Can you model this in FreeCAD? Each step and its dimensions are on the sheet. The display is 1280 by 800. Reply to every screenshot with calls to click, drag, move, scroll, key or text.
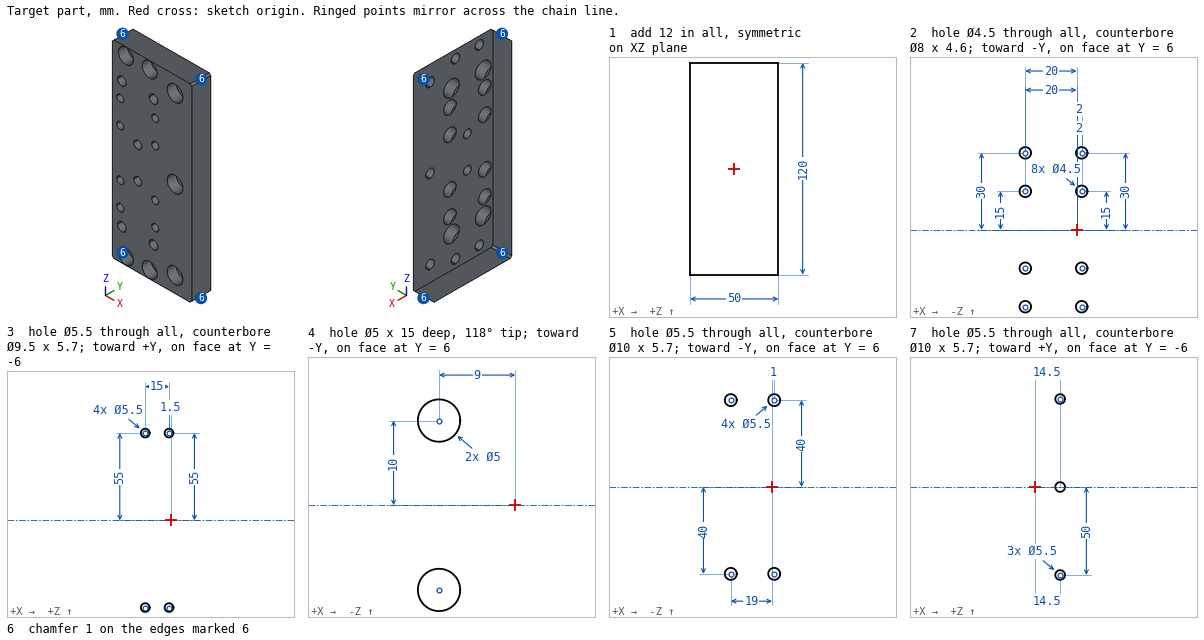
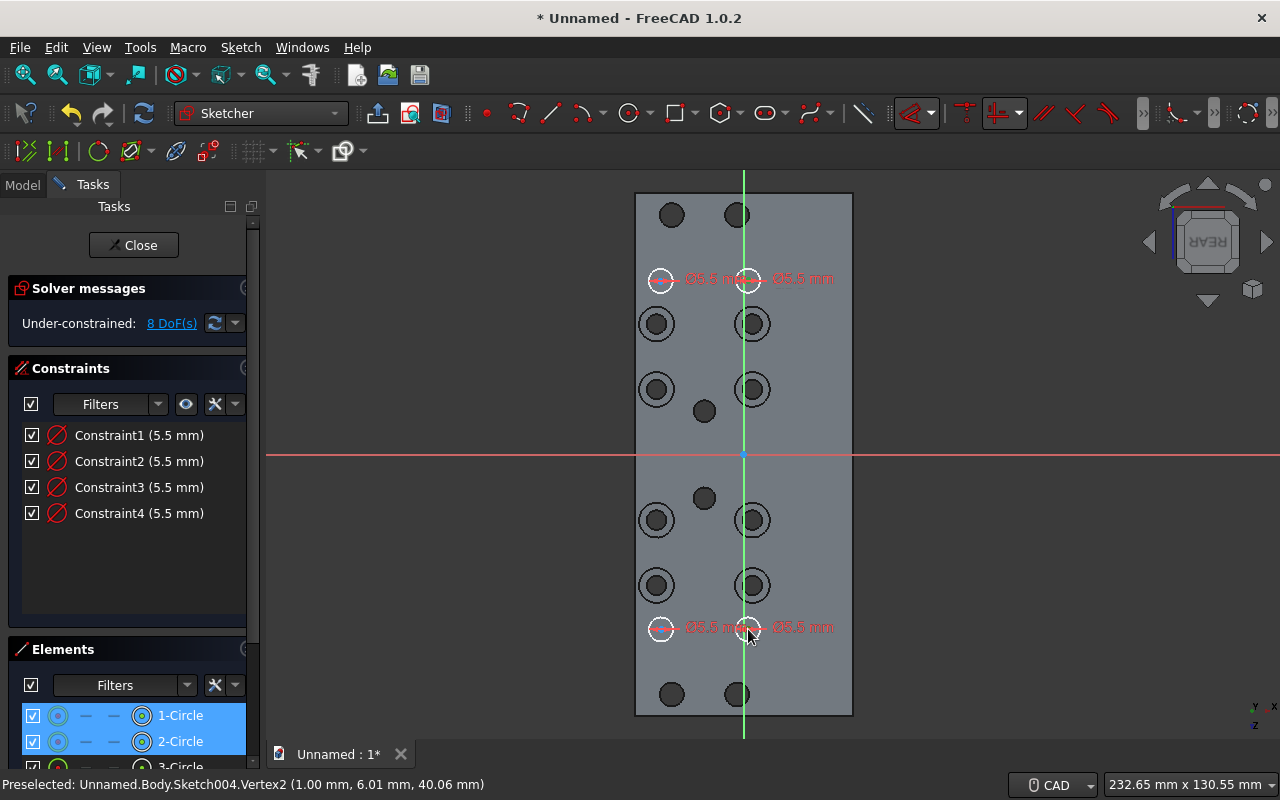
click(353, 455)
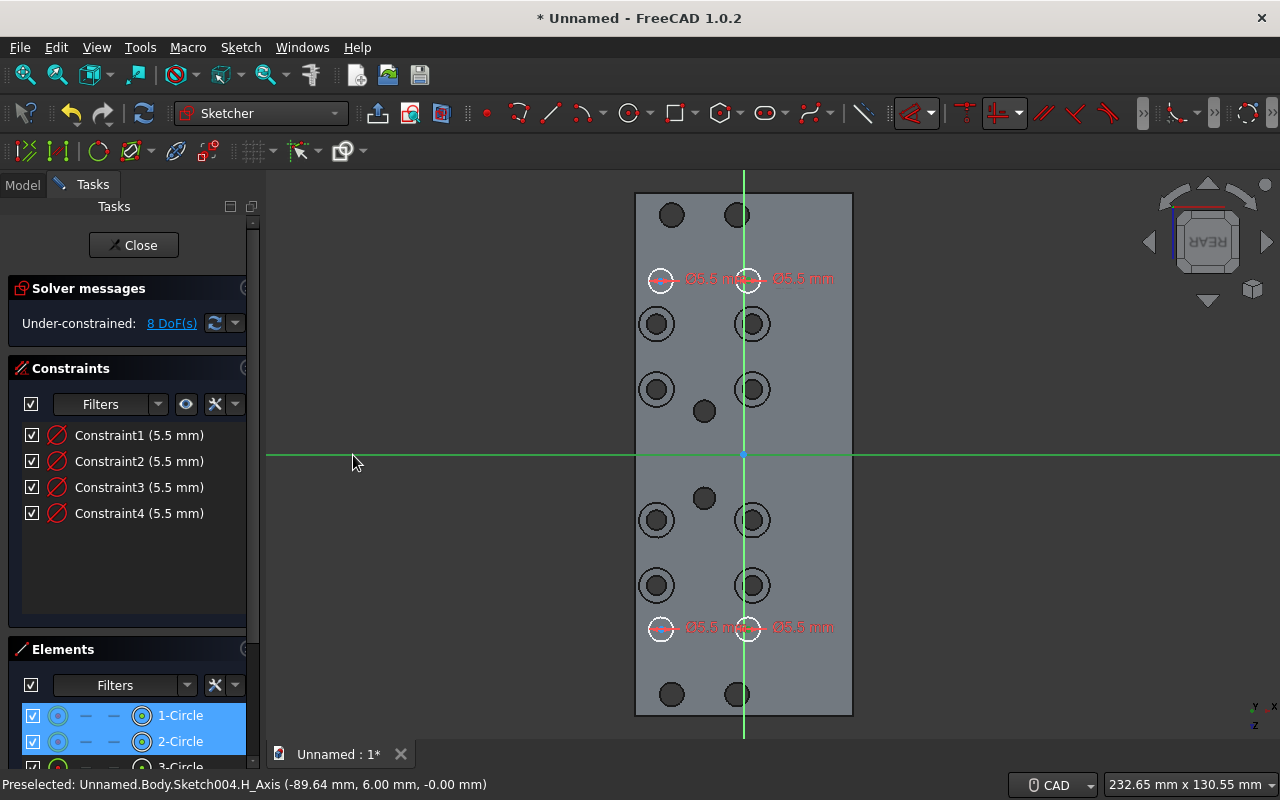
key(s)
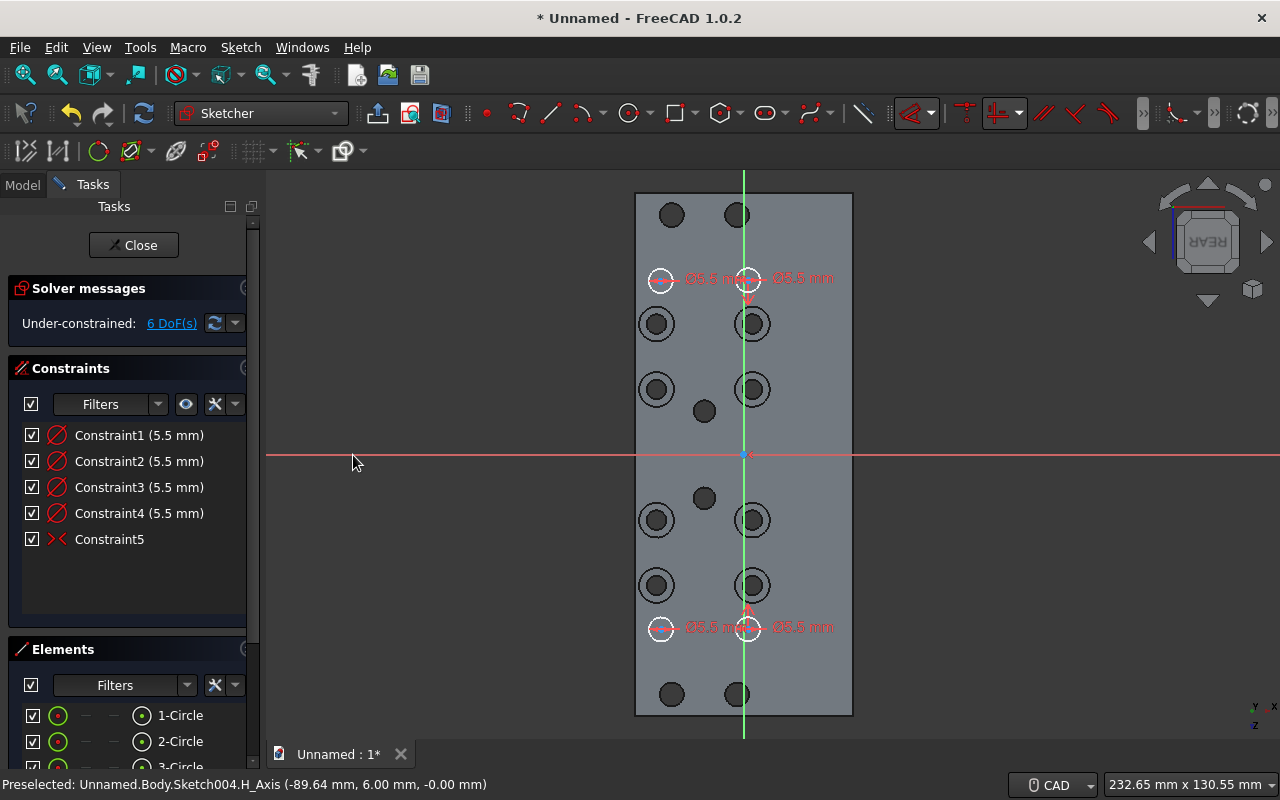
click(661, 629)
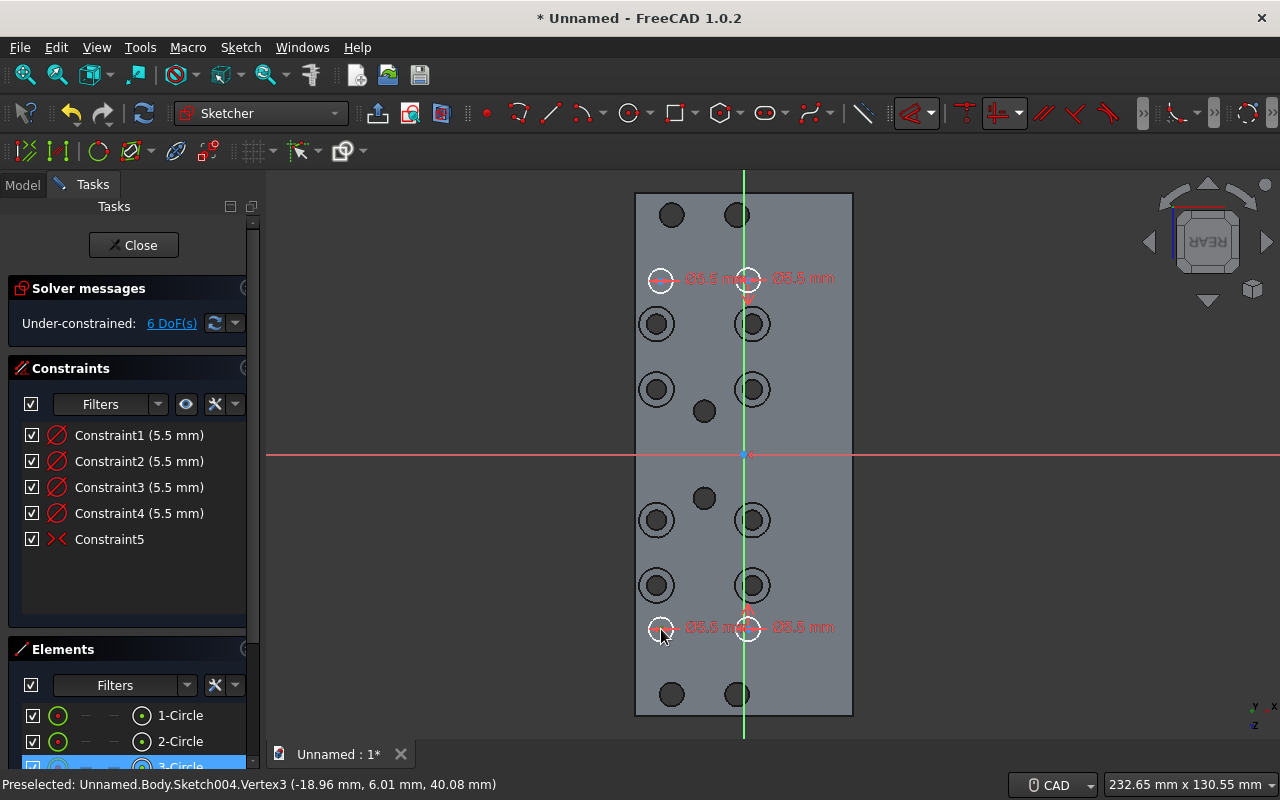
click(661, 281)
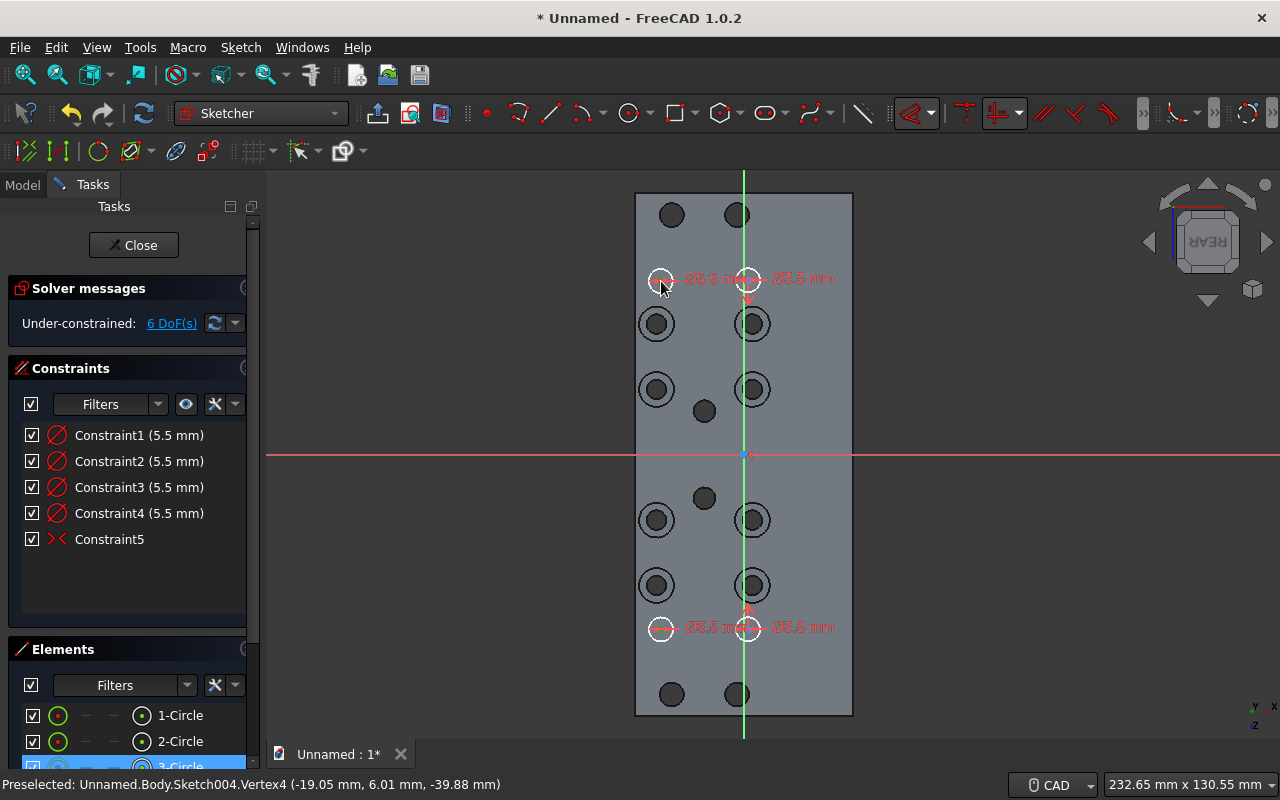
click(353, 455)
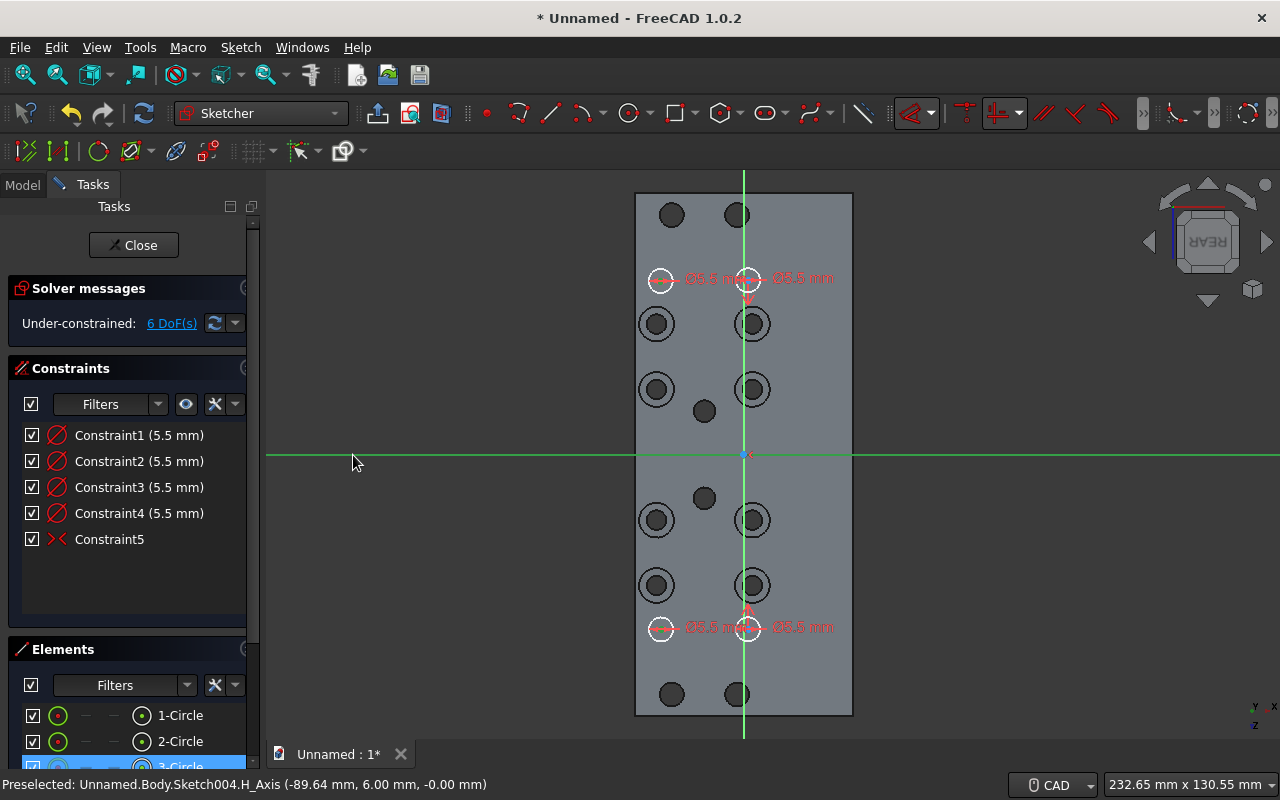
key(s)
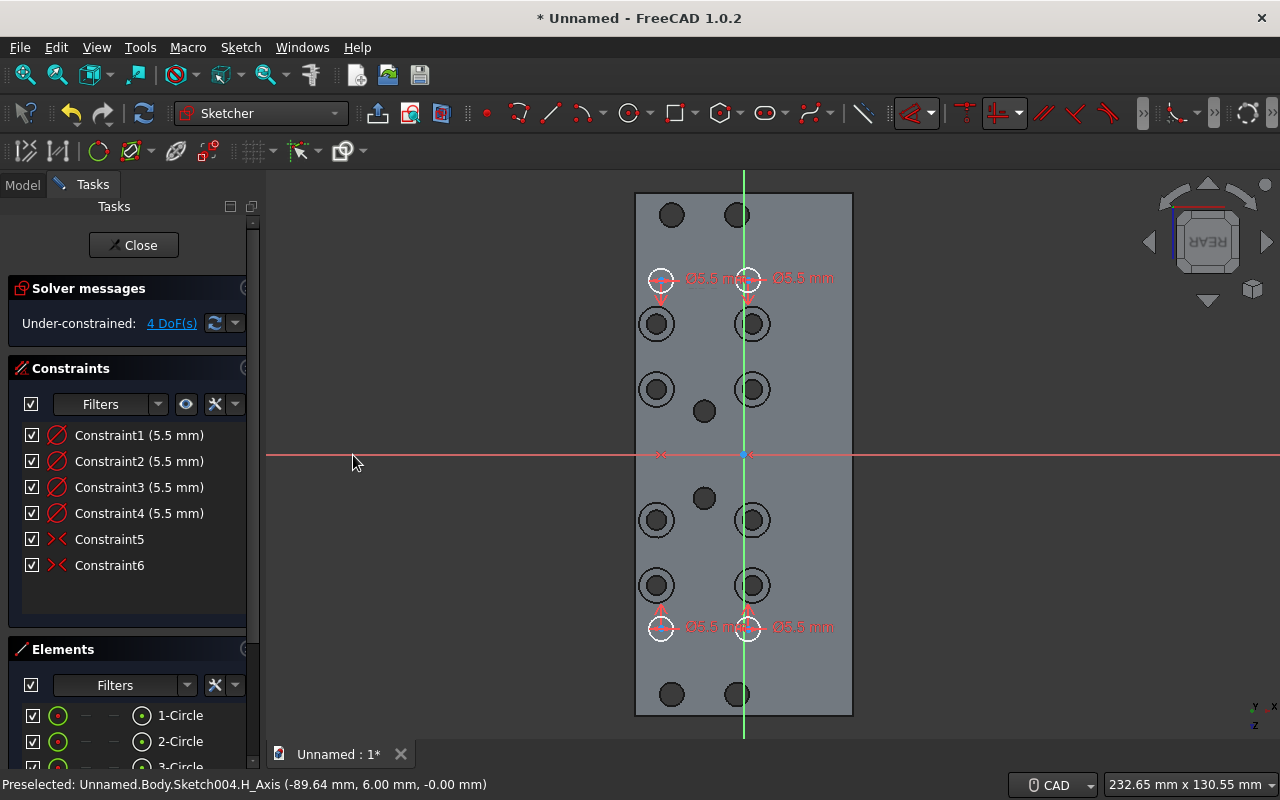
scroll(748, 280, up, 12)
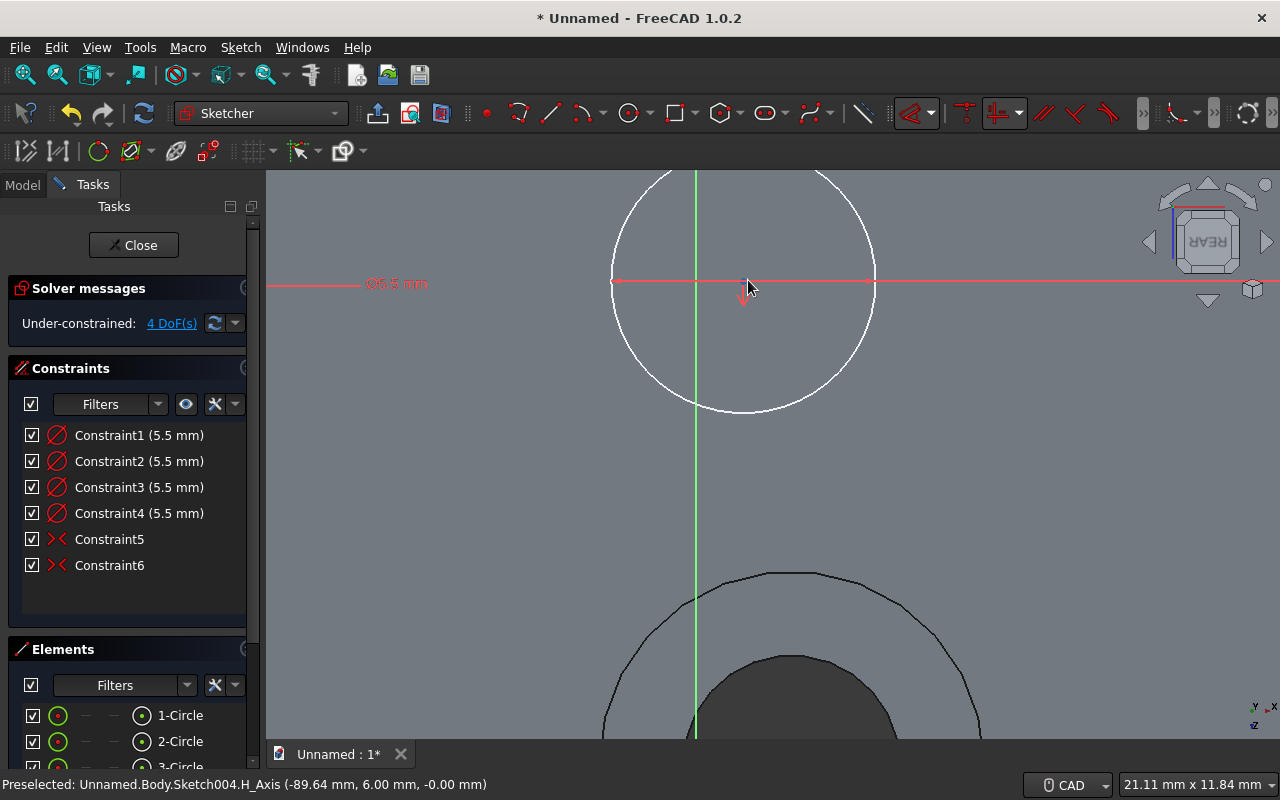
click(743, 281)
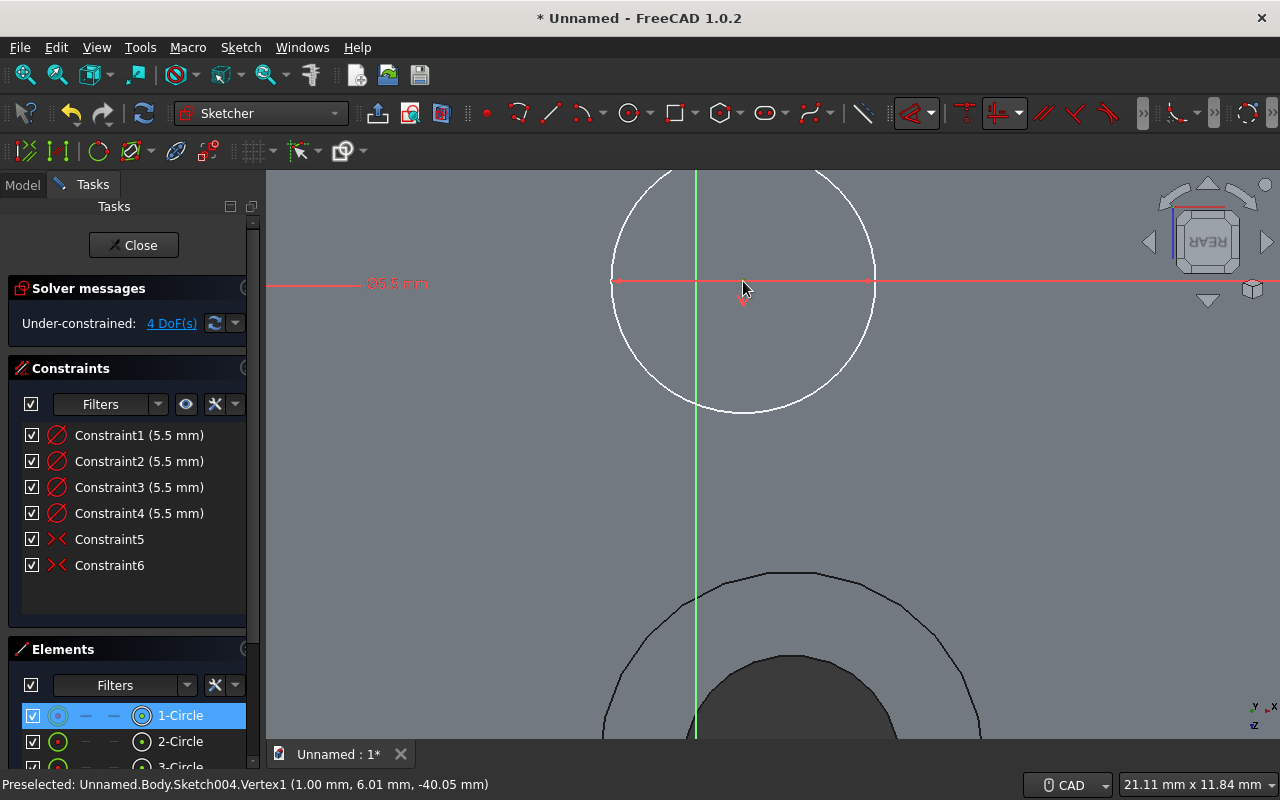
click(934, 114)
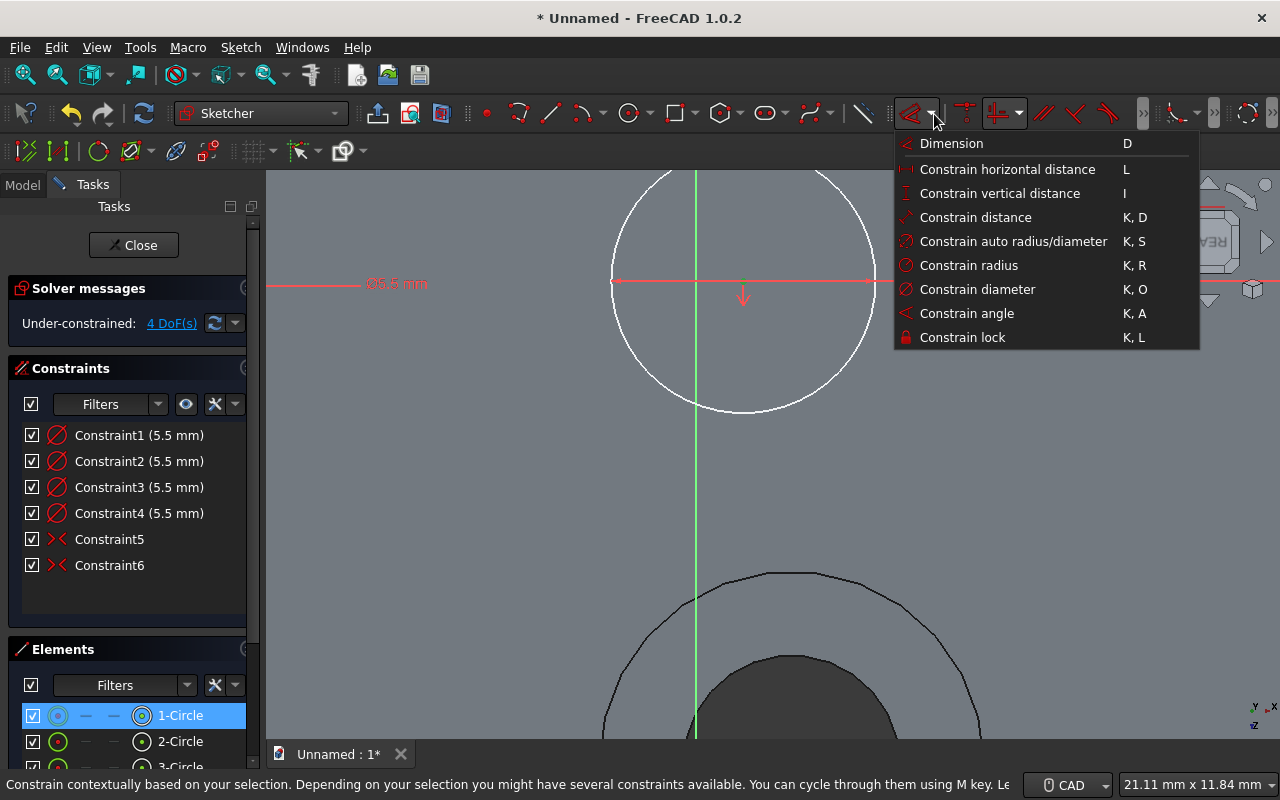
click(1047, 169)